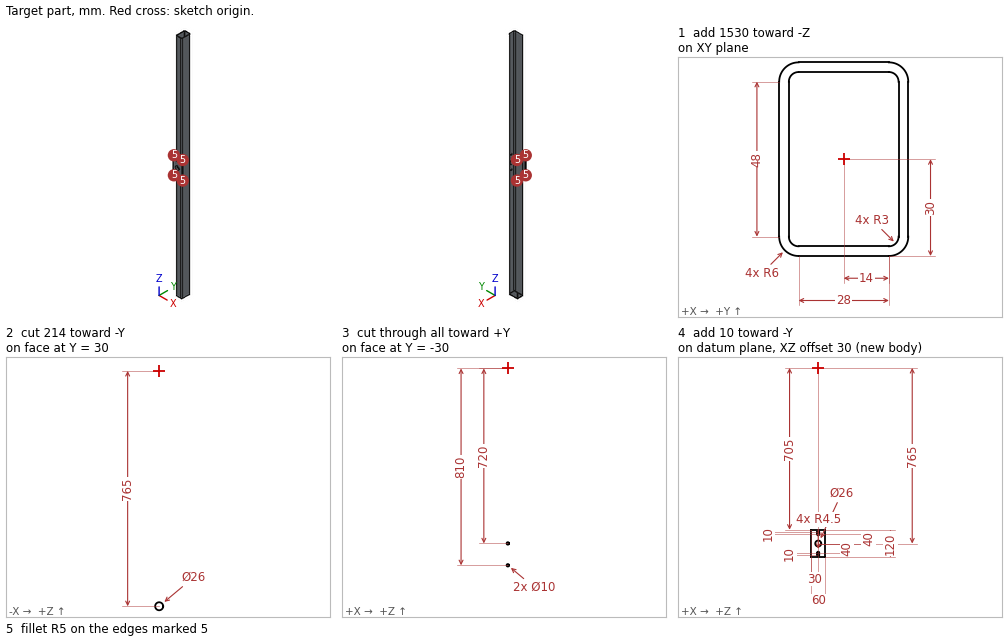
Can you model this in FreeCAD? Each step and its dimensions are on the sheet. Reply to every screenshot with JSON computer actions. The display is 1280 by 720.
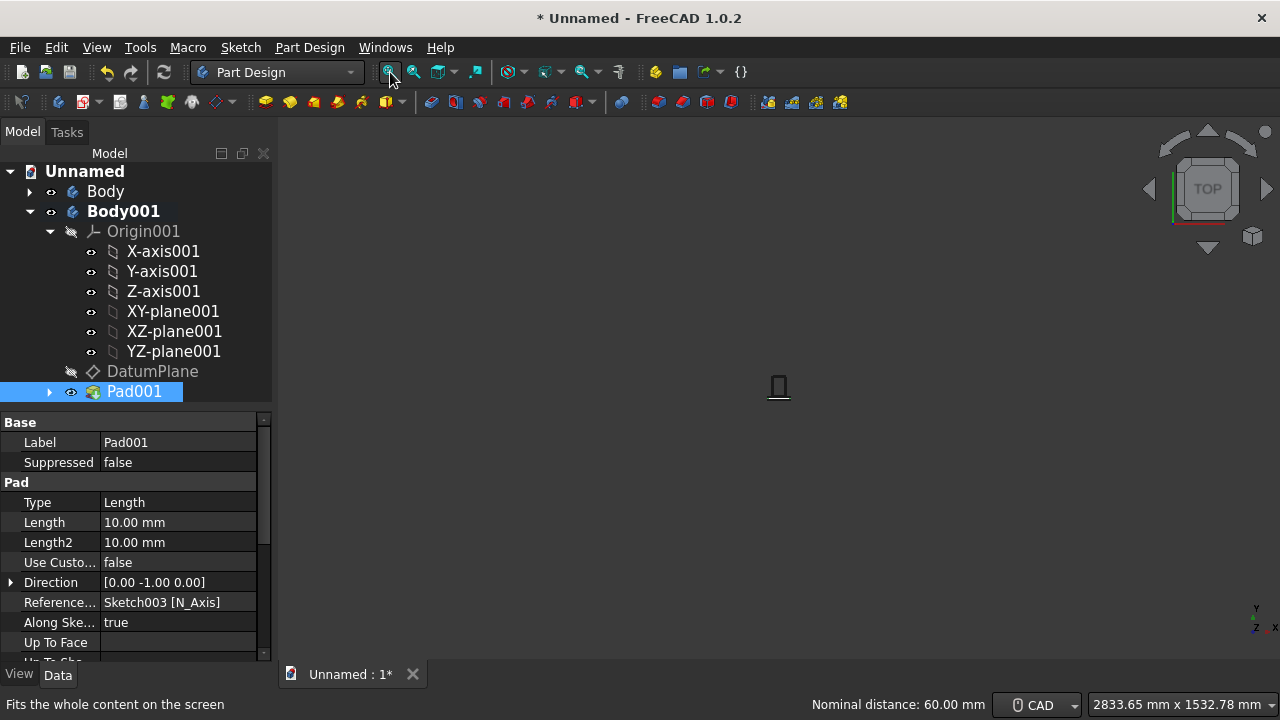
{"action": "key", "text": "0"}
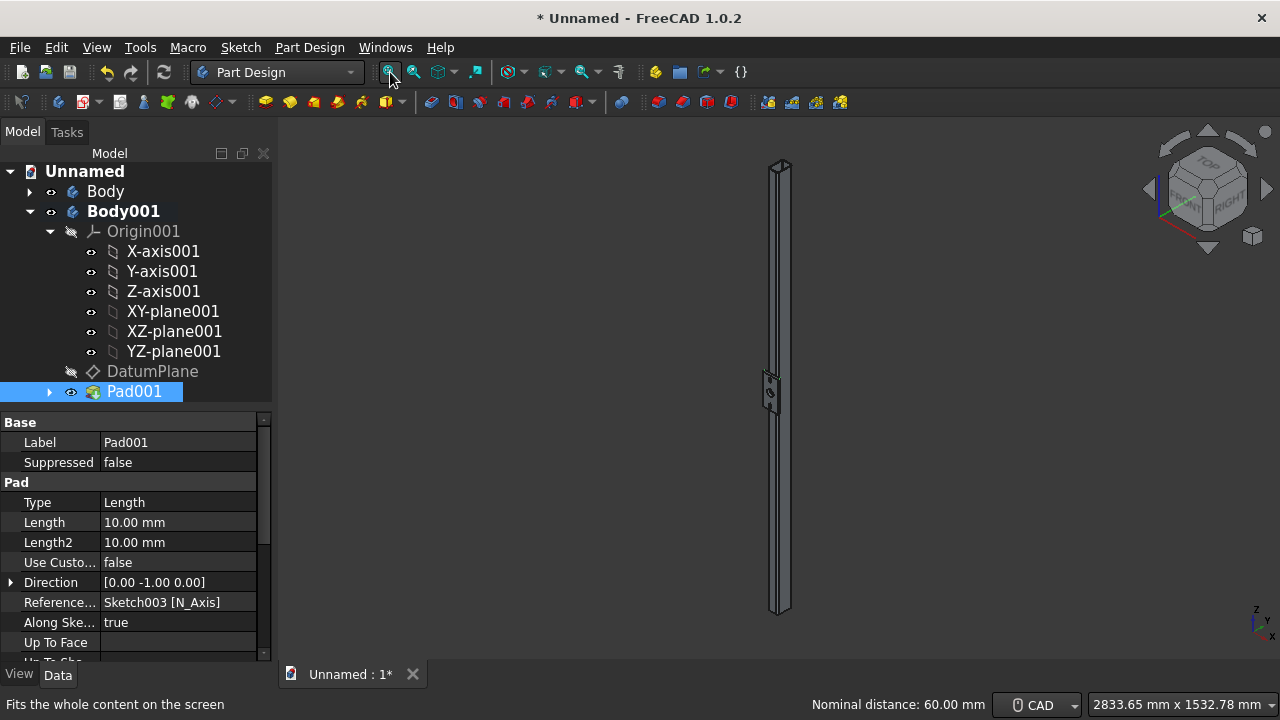
{"action": "left_click", "coordinate": [390, 72]}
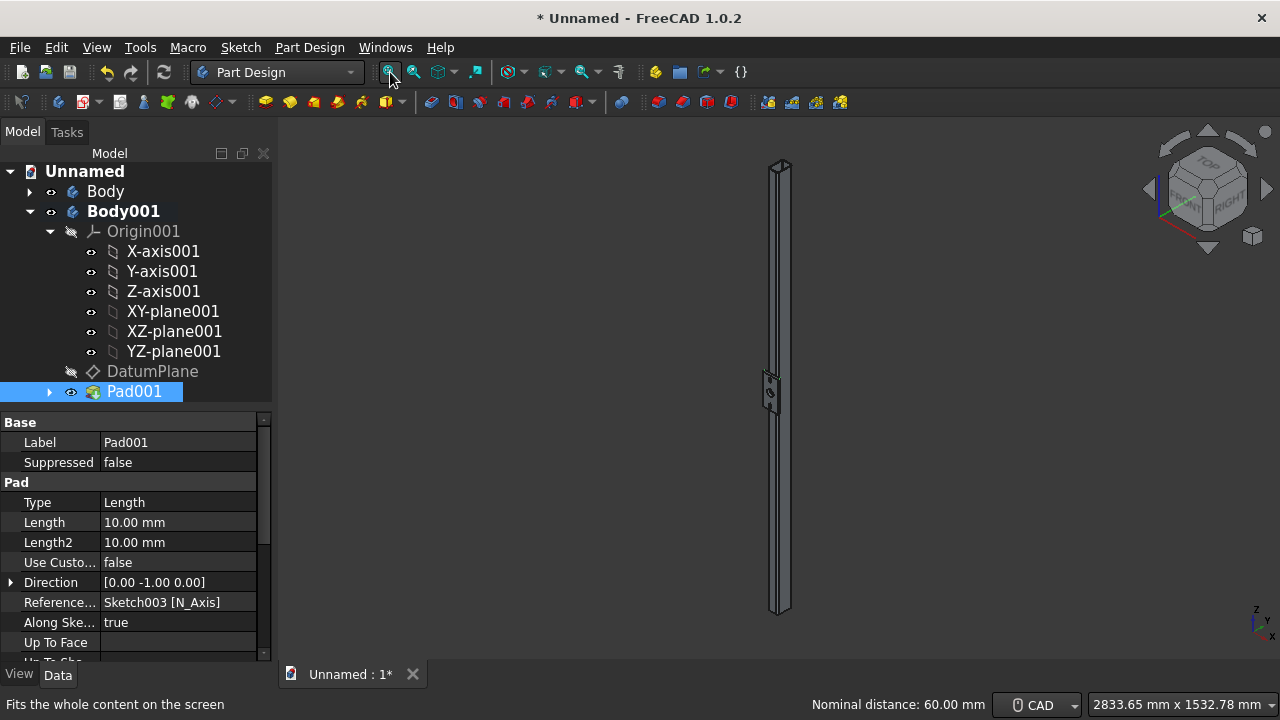
{"action": "scroll", "coordinate": [779, 413], "scroll_direction": "up", "scroll_amount": 13}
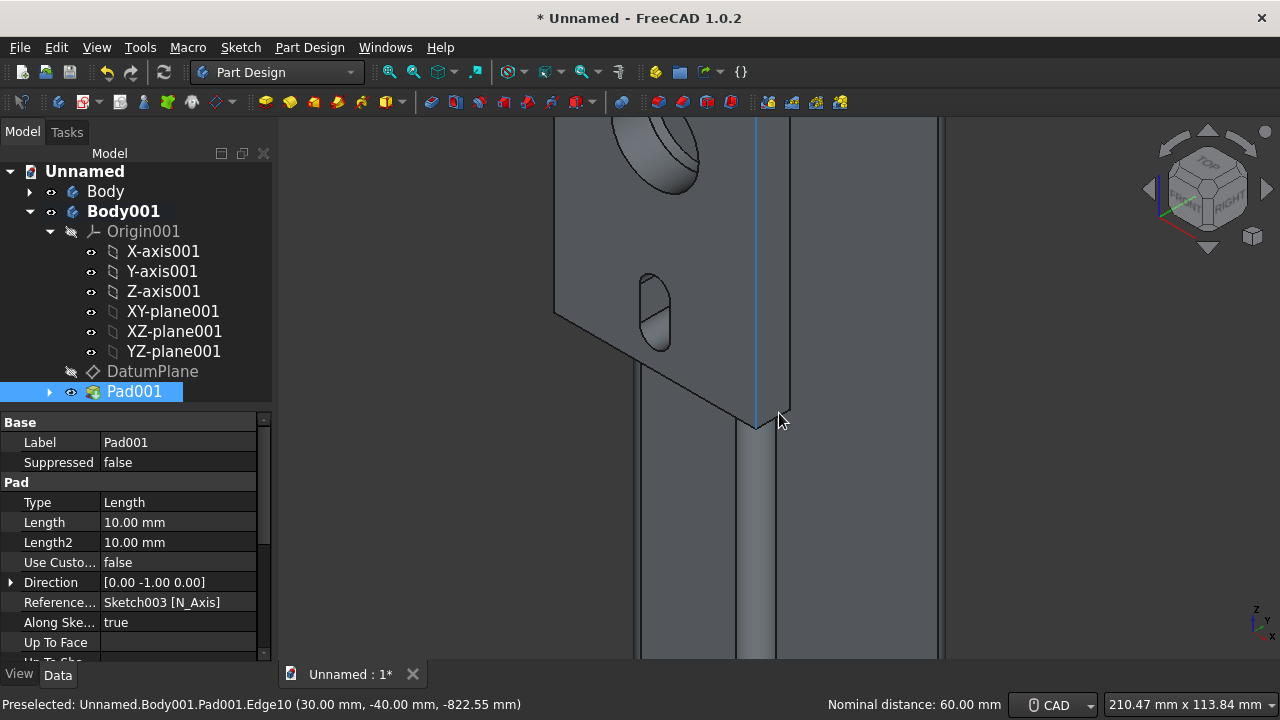
{"action": "left_click", "coordinate": [390, 72]}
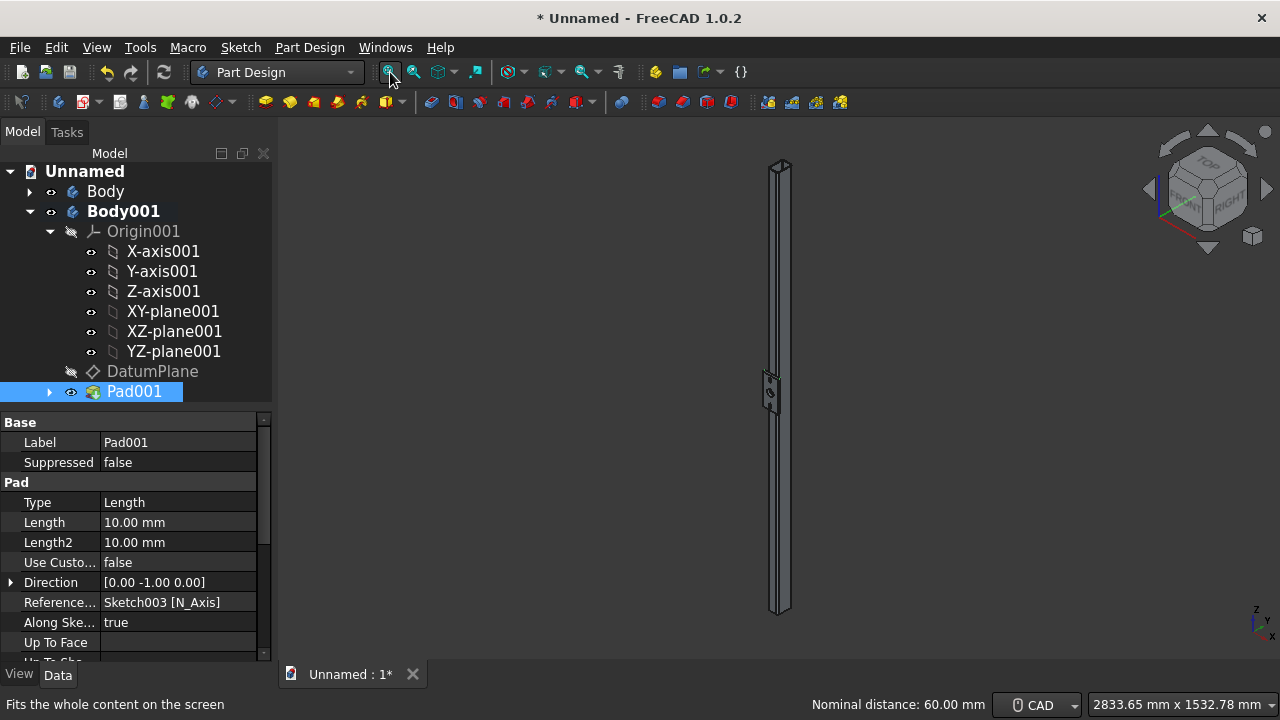
{"action": "key", "text": "1"}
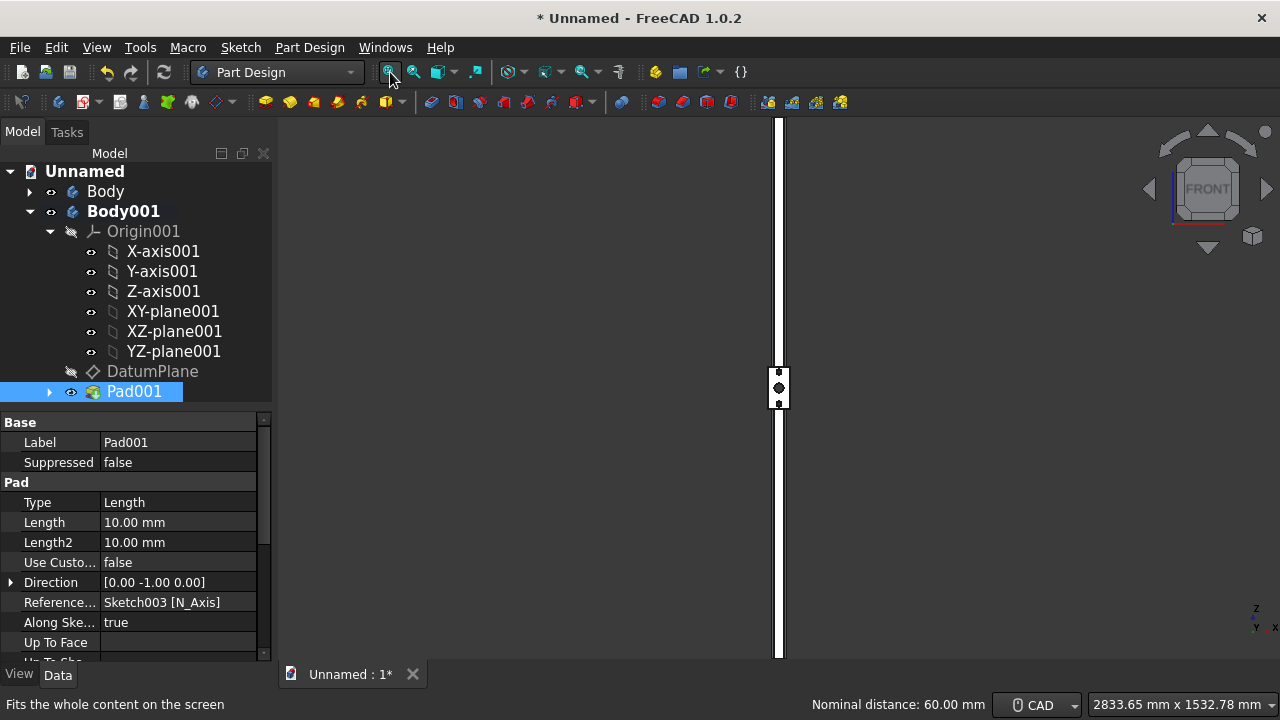
{"action": "left_click", "coordinate": [390, 72]}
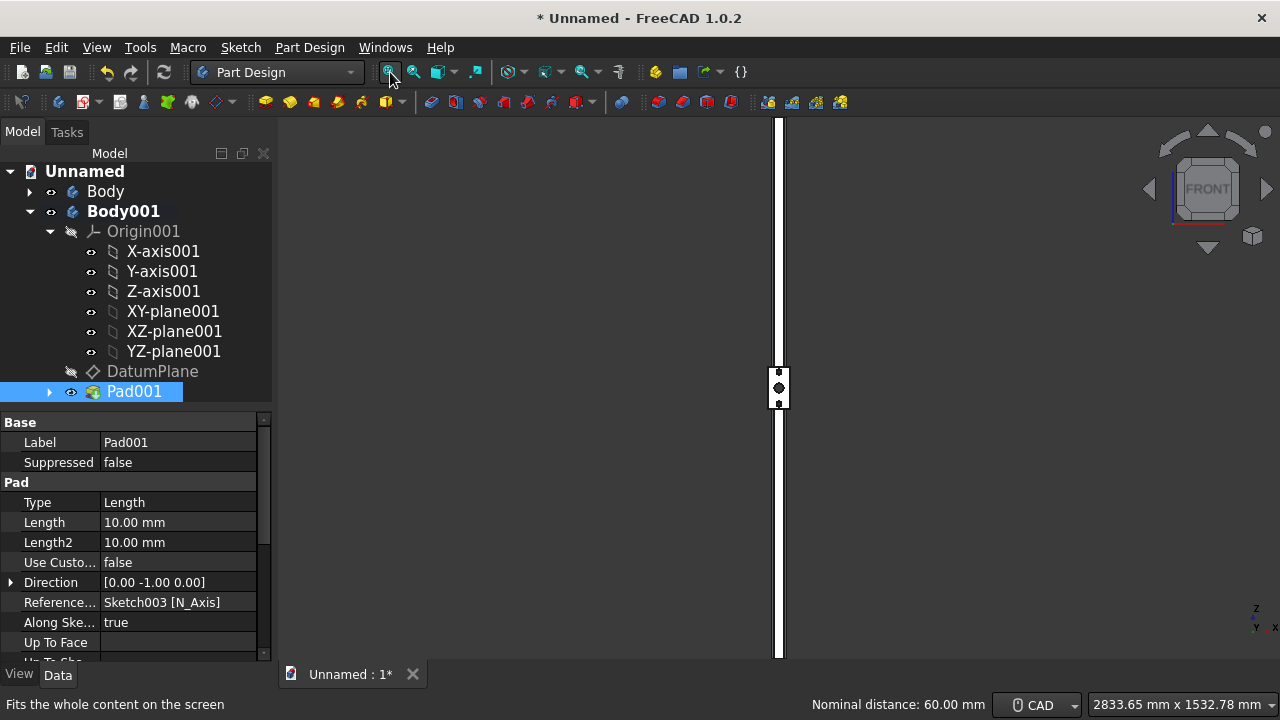
{"action": "scroll", "coordinate": [790, 408], "scroll_direction": "up", "scroll_amount": 13}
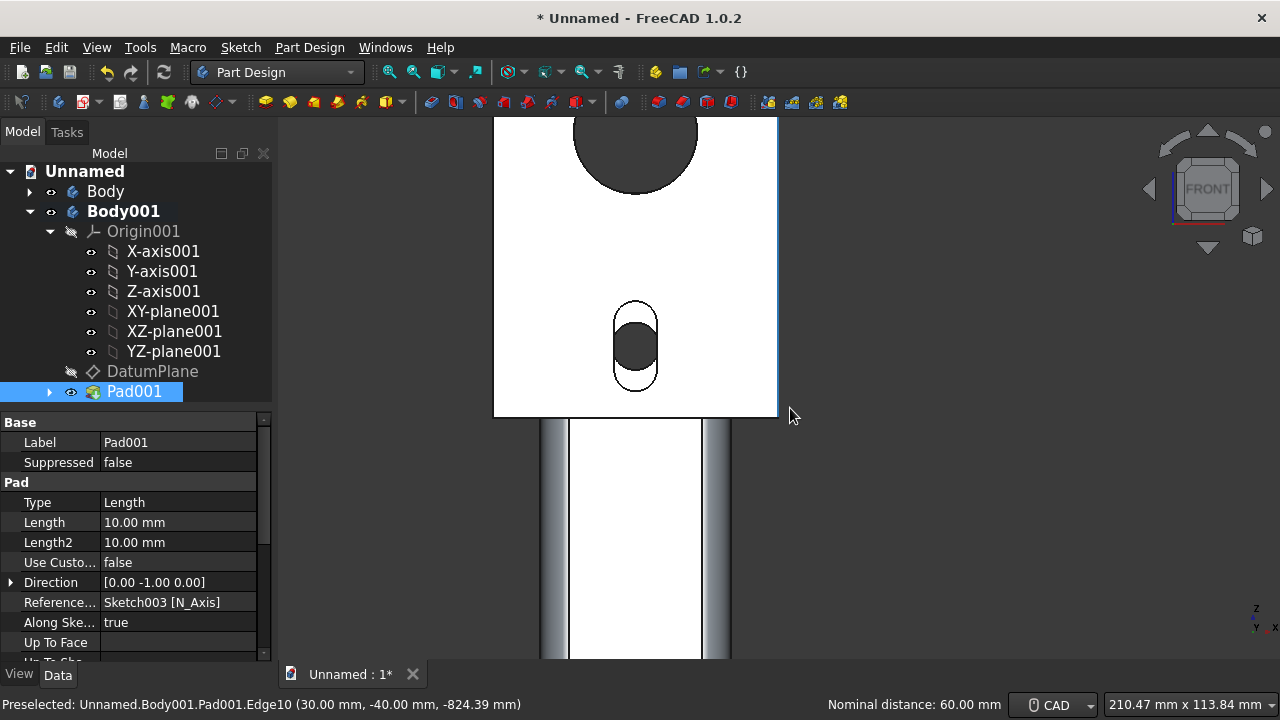
{"action": "left_click", "coordinate": [390, 72]}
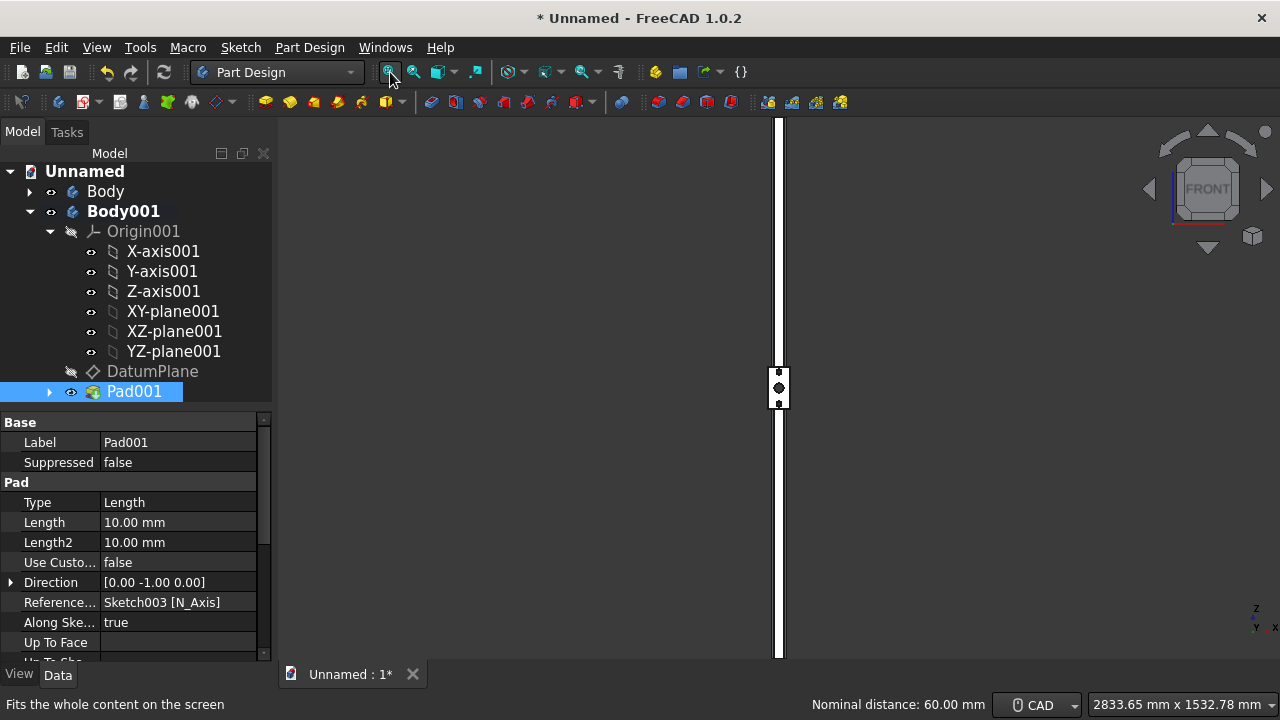
{"action": "key", "text": "3"}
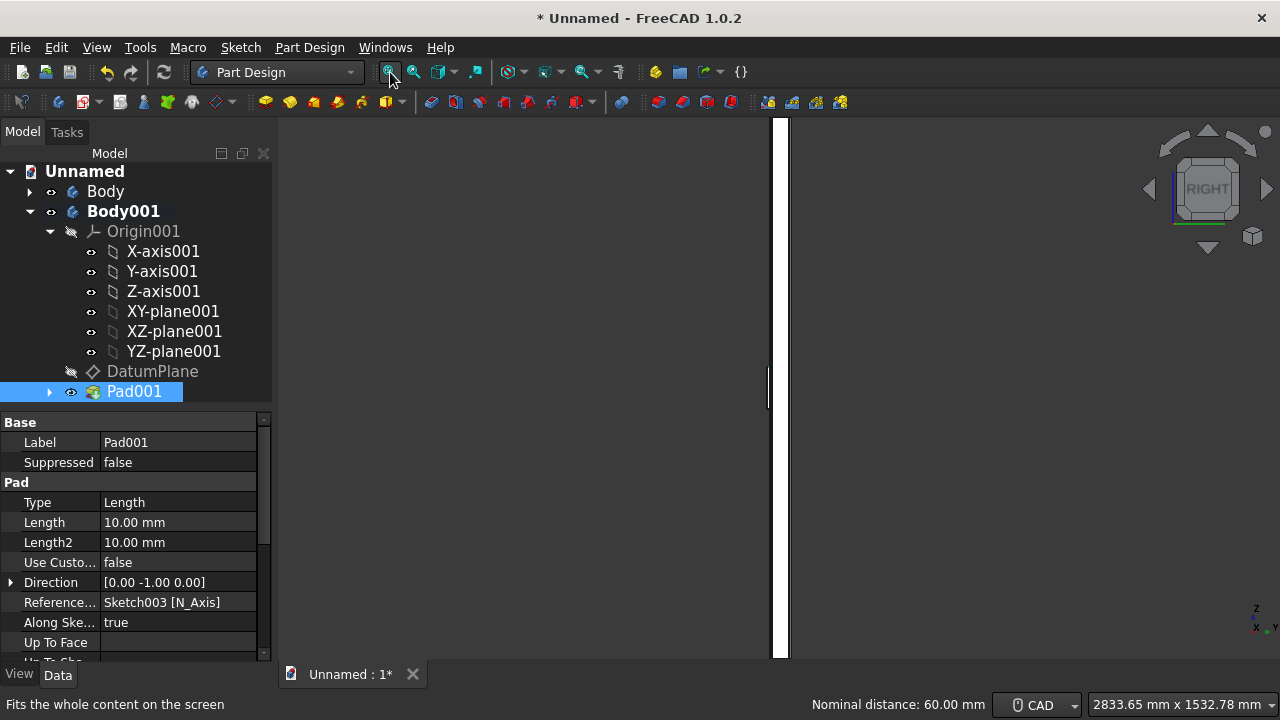
{"action": "left_click", "coordinate": [390, 72]}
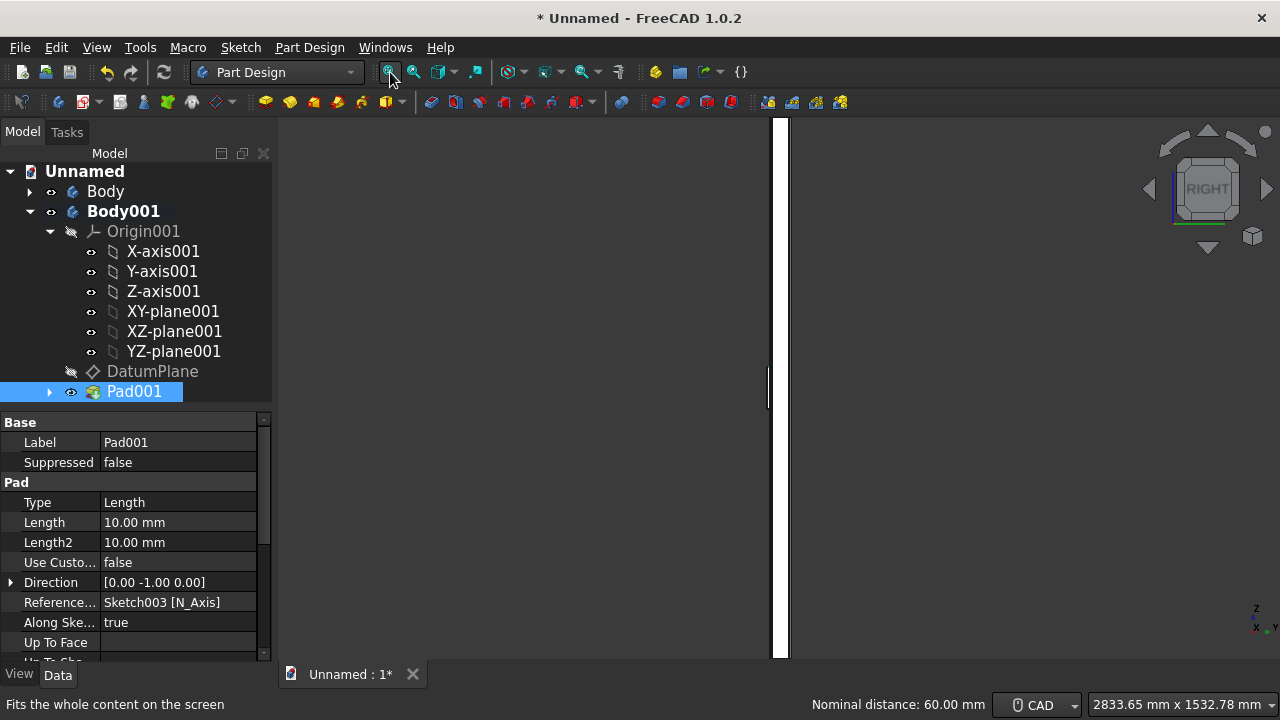
{"action": "scroll", "coordinate": [768, 408], "scroll_direction": "up", "scroll_amount": 13}